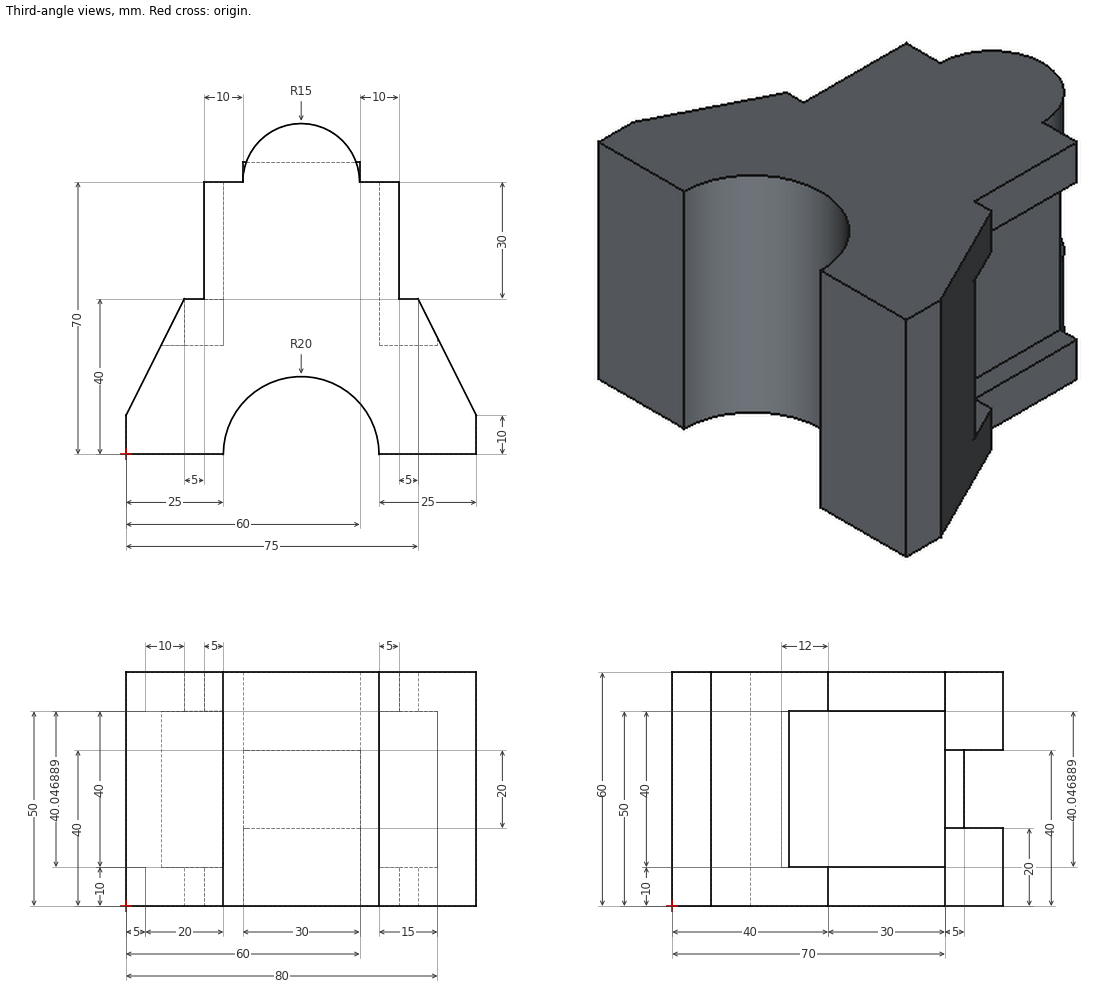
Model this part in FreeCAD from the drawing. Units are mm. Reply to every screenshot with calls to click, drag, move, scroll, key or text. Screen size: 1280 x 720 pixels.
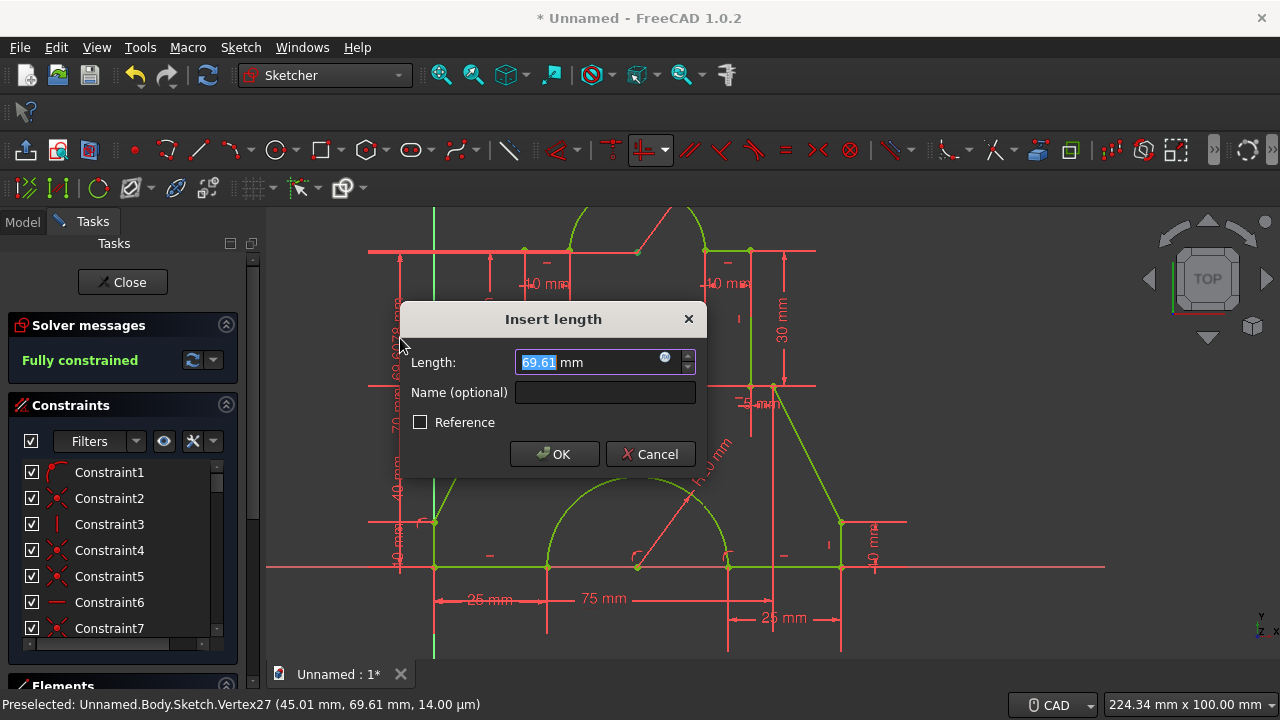
text(70)
key(Return)
key(Escape)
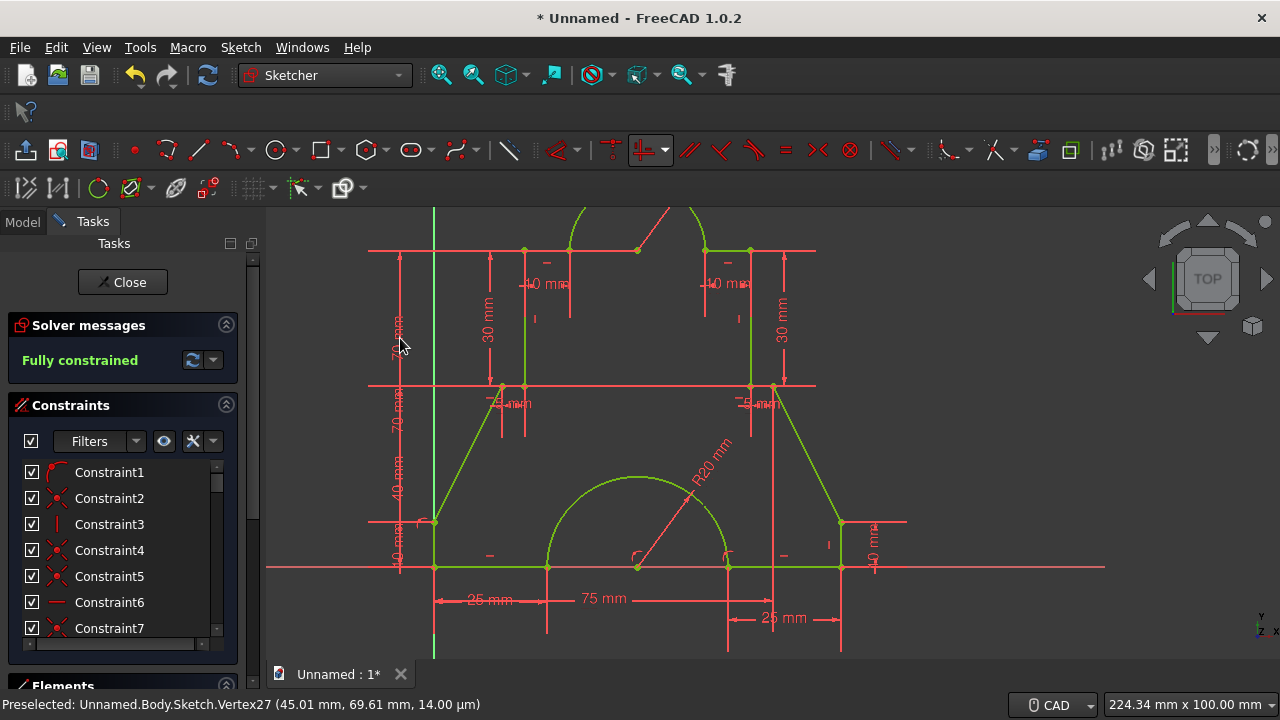
click(123, 282)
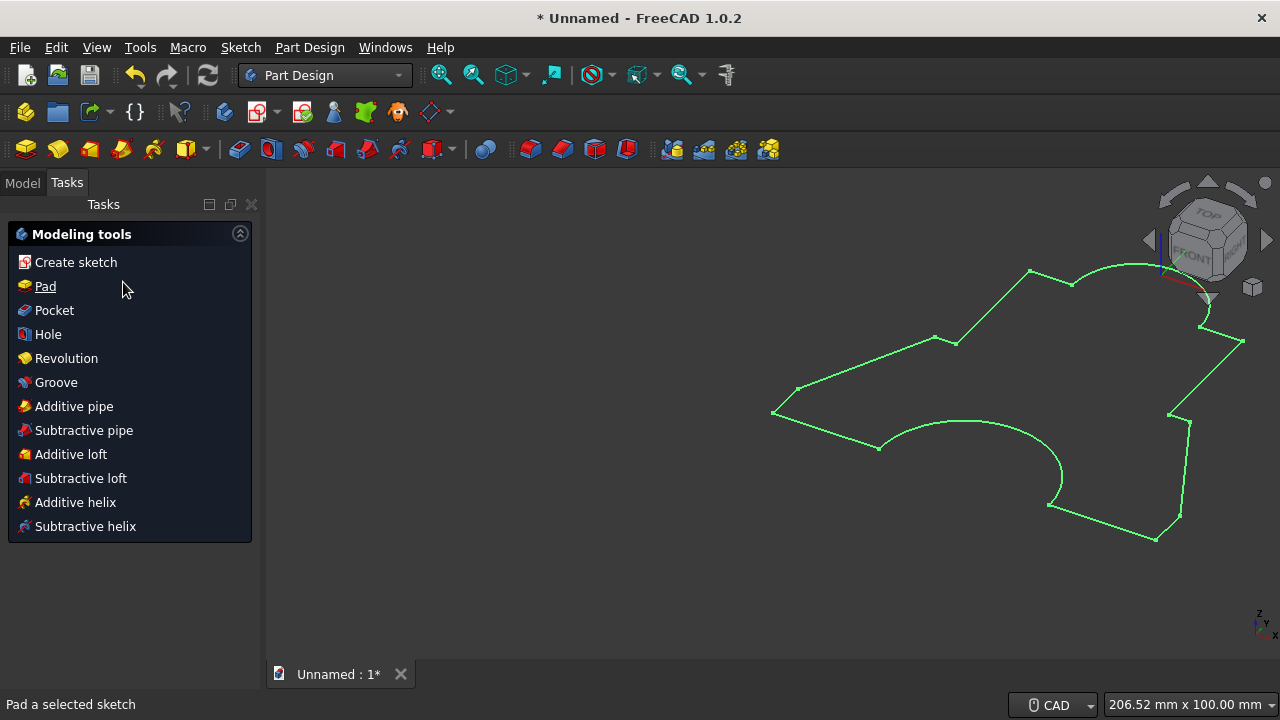
click(26, 150)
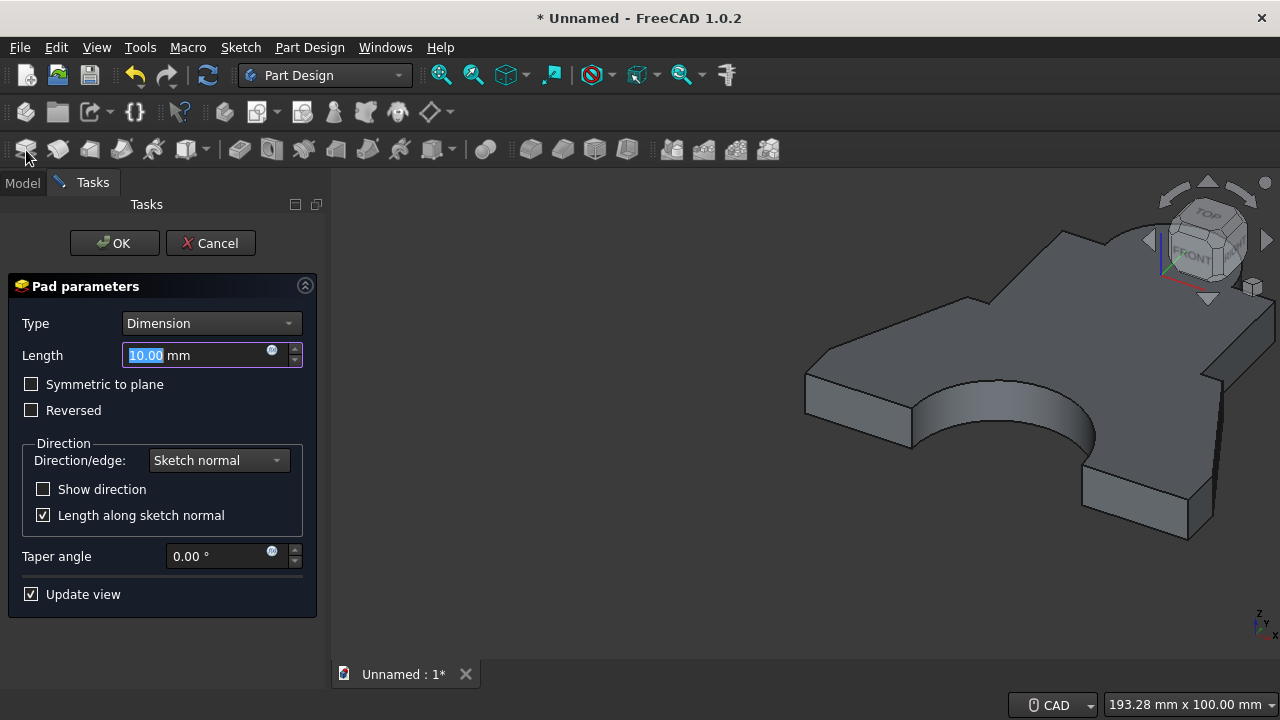
text(60)
key(Tab)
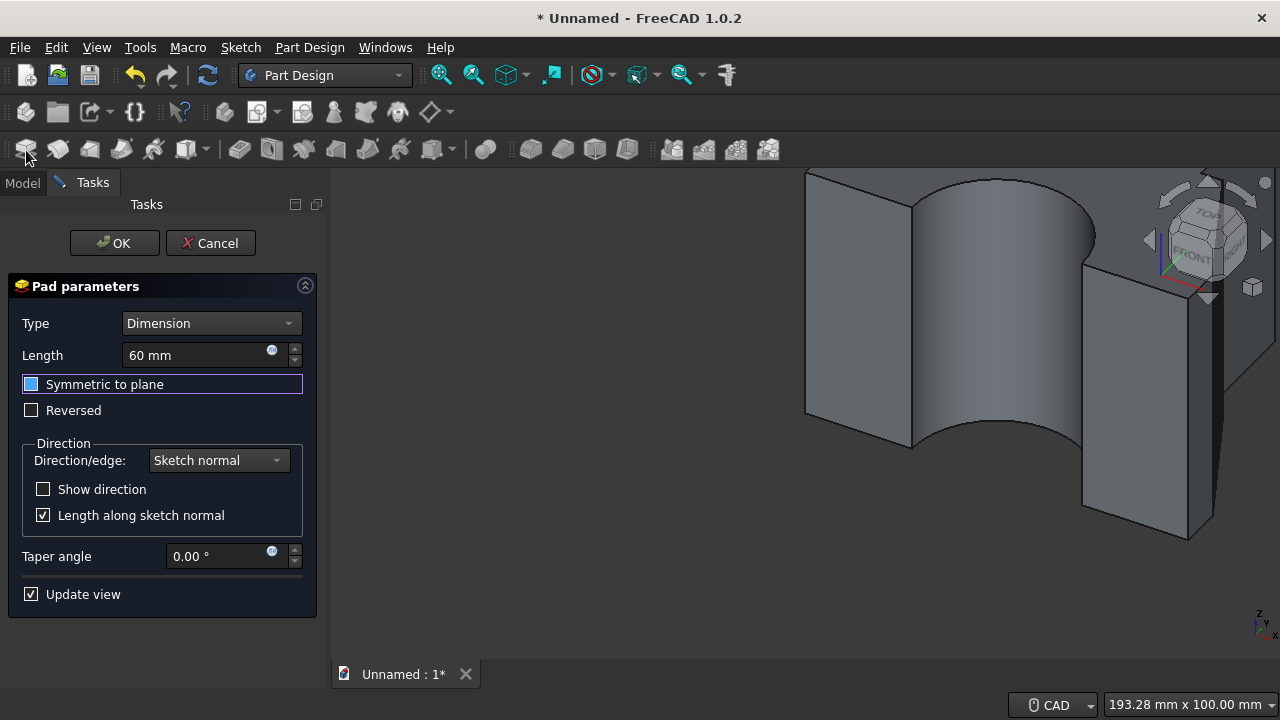
click(115, 243)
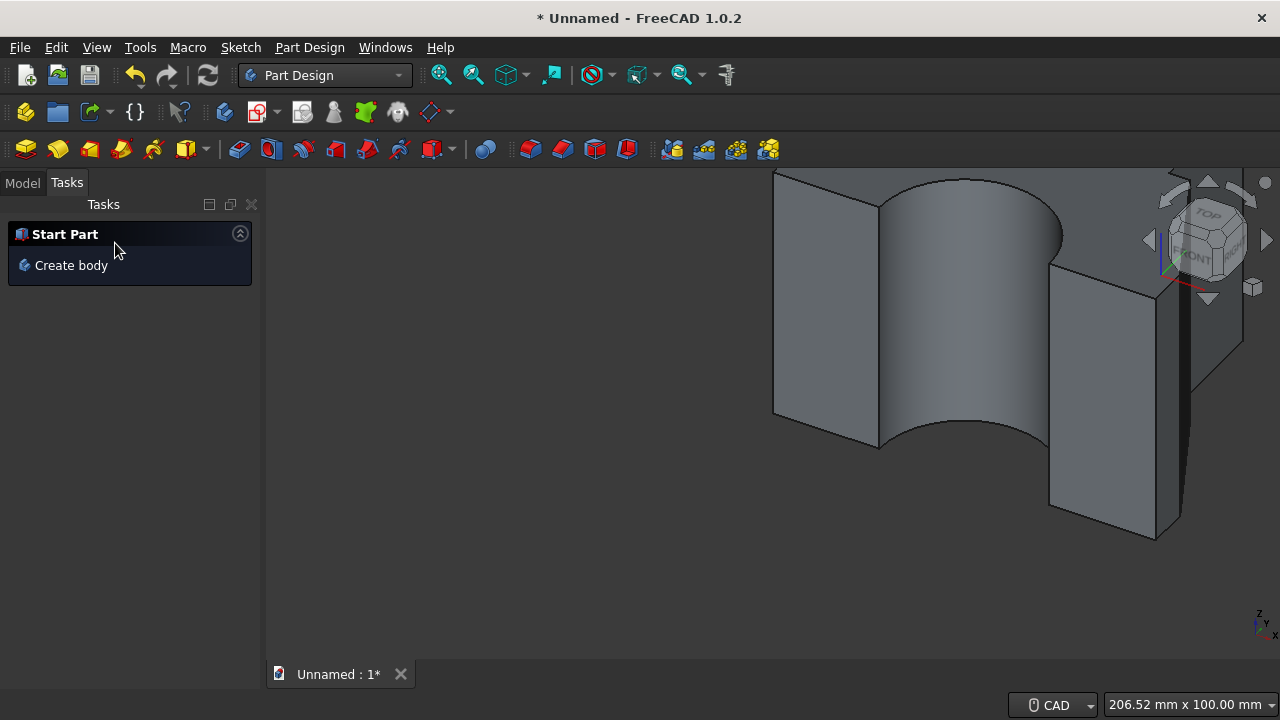
click(442, 76)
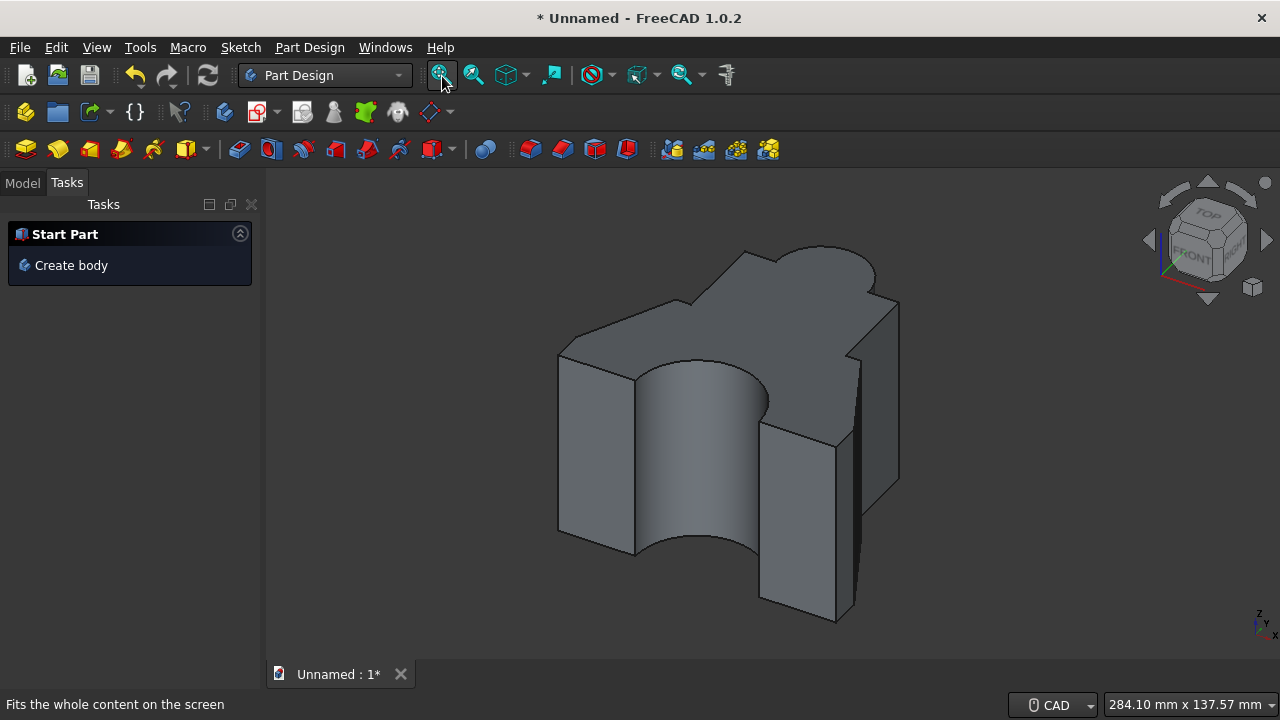
key(6)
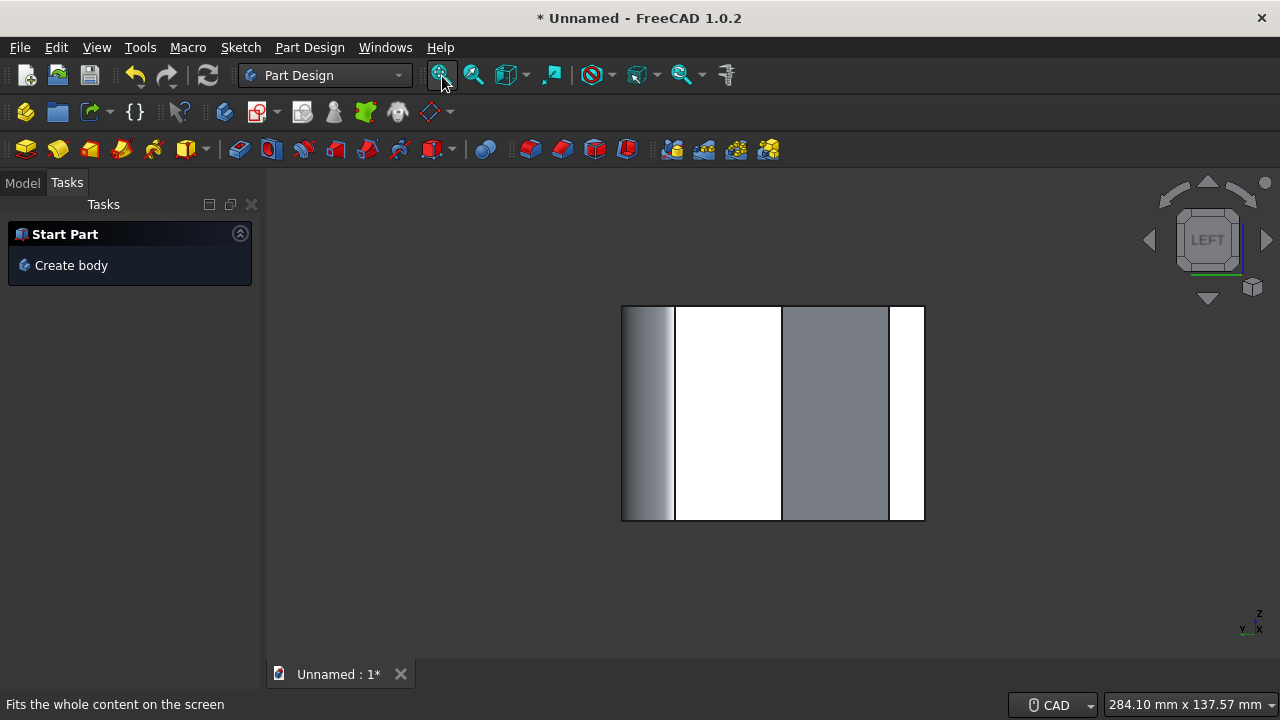
key(v)
key(f)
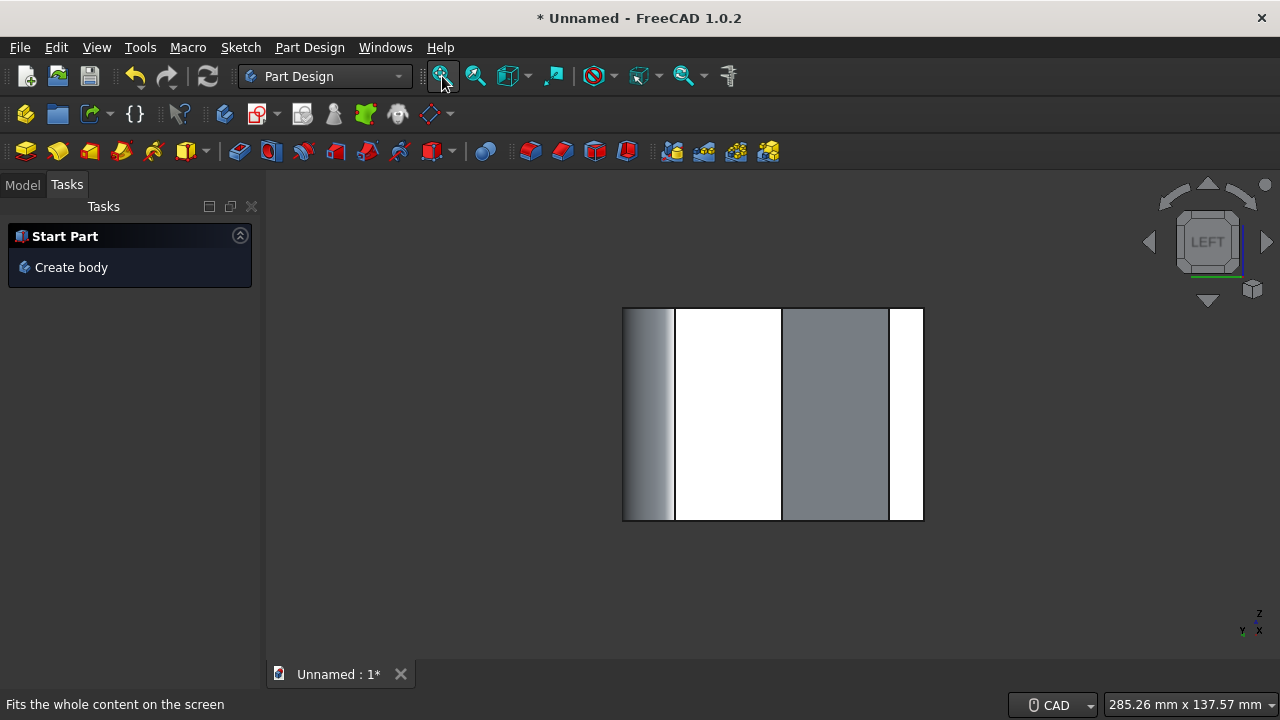
click(729, 383)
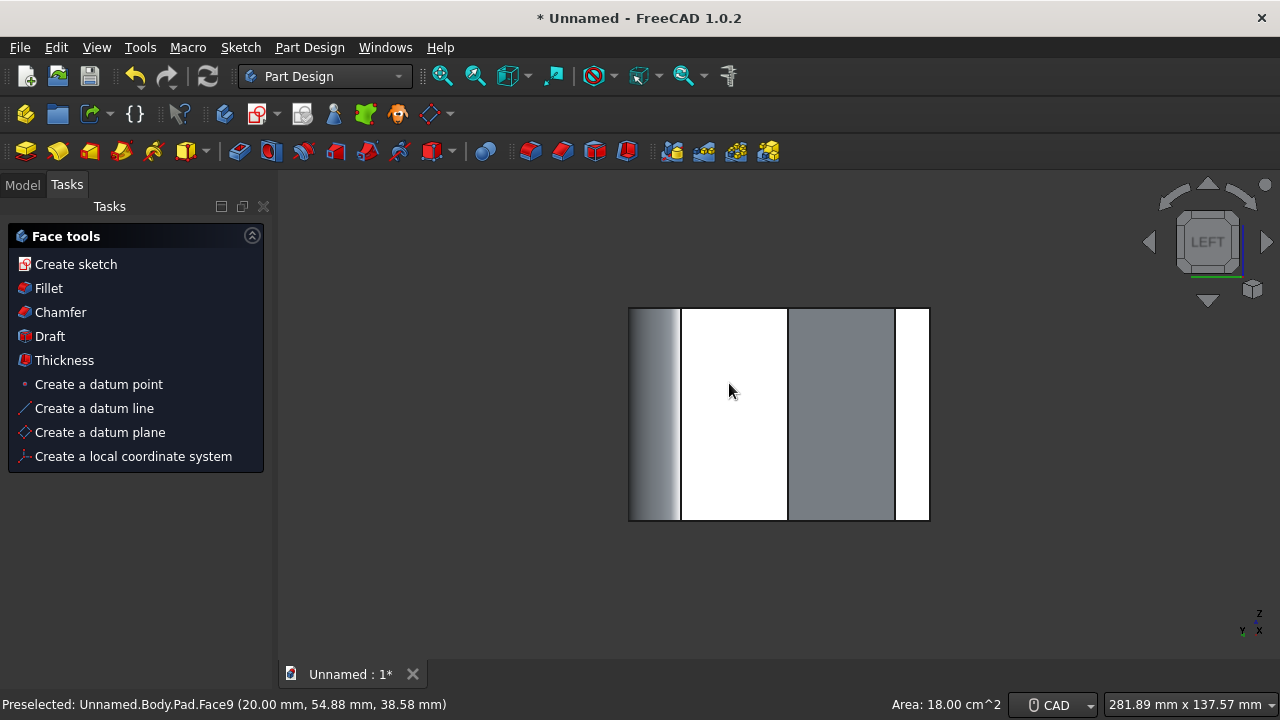
click(258, 114)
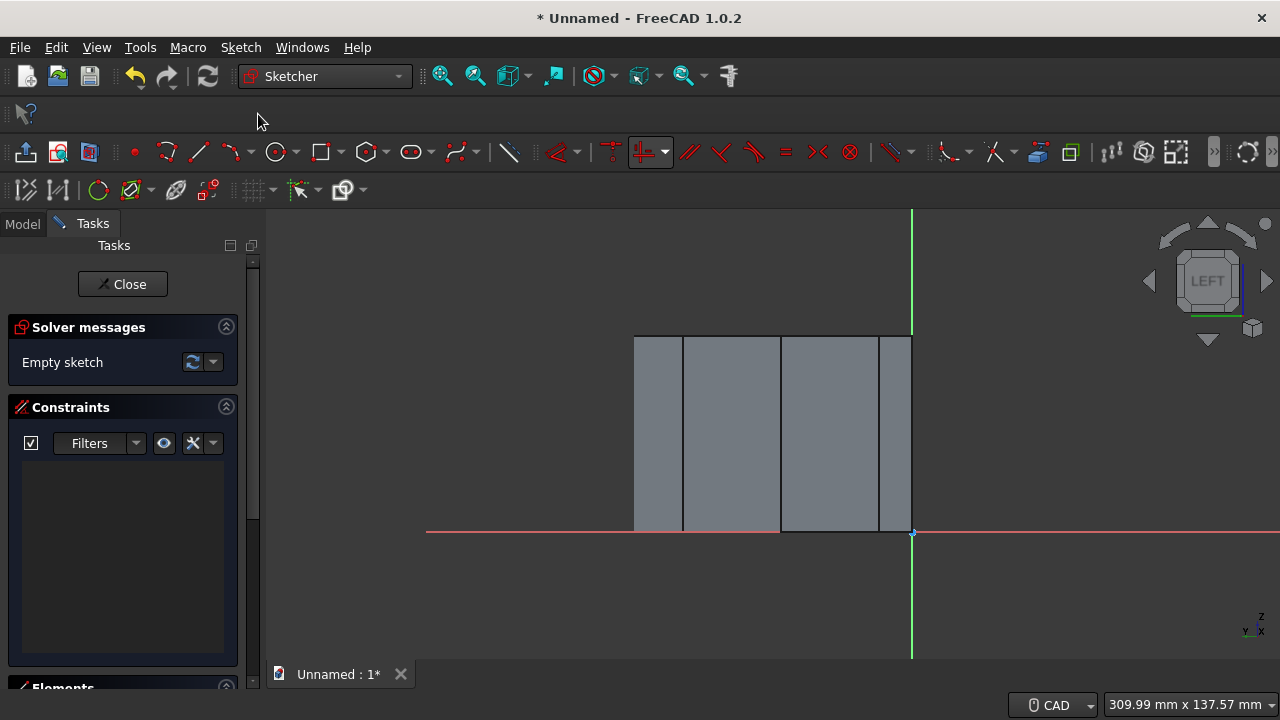
scroll(911, 470, up, 3)